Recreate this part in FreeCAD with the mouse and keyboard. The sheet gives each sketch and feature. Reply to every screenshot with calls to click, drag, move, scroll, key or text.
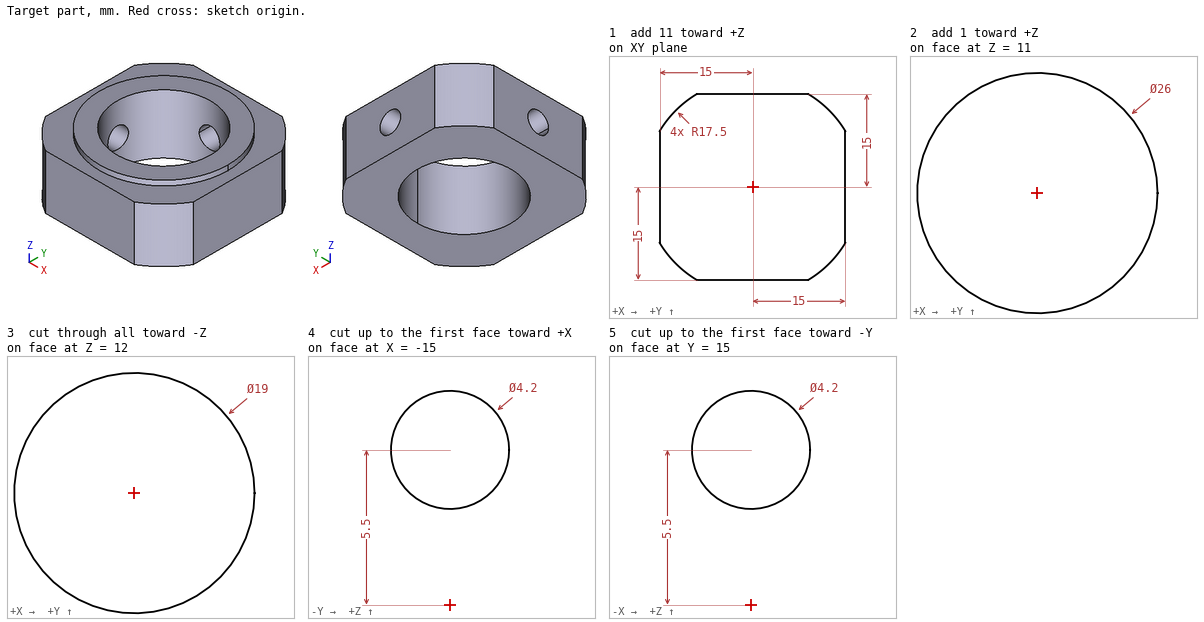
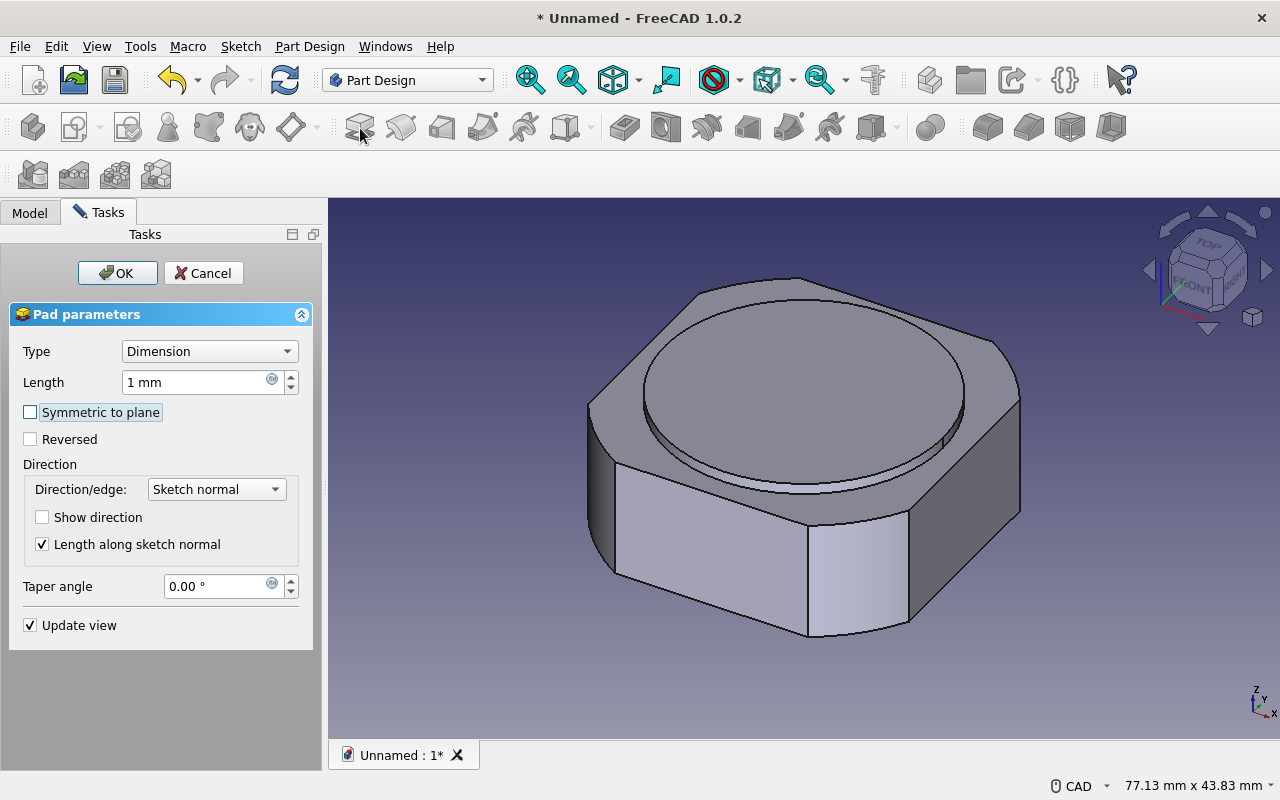
click(118, 273)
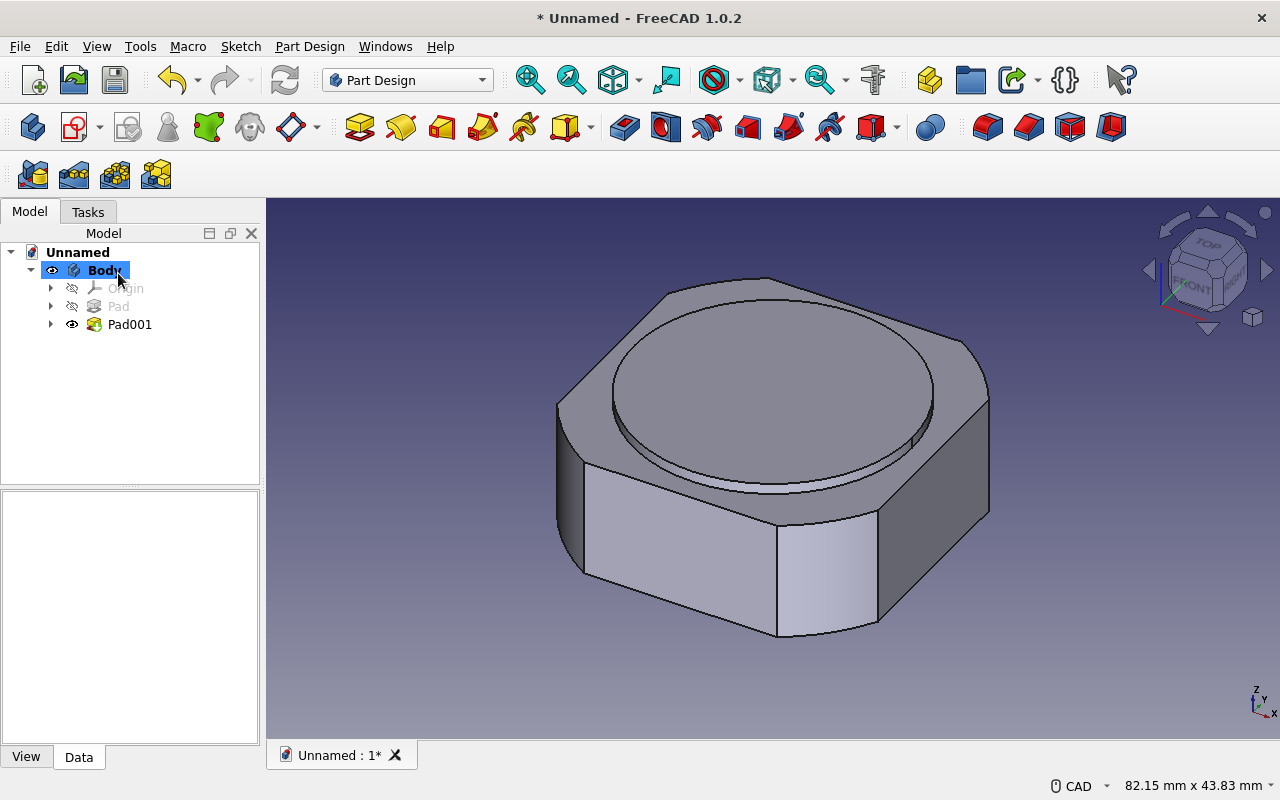
click(773, 391)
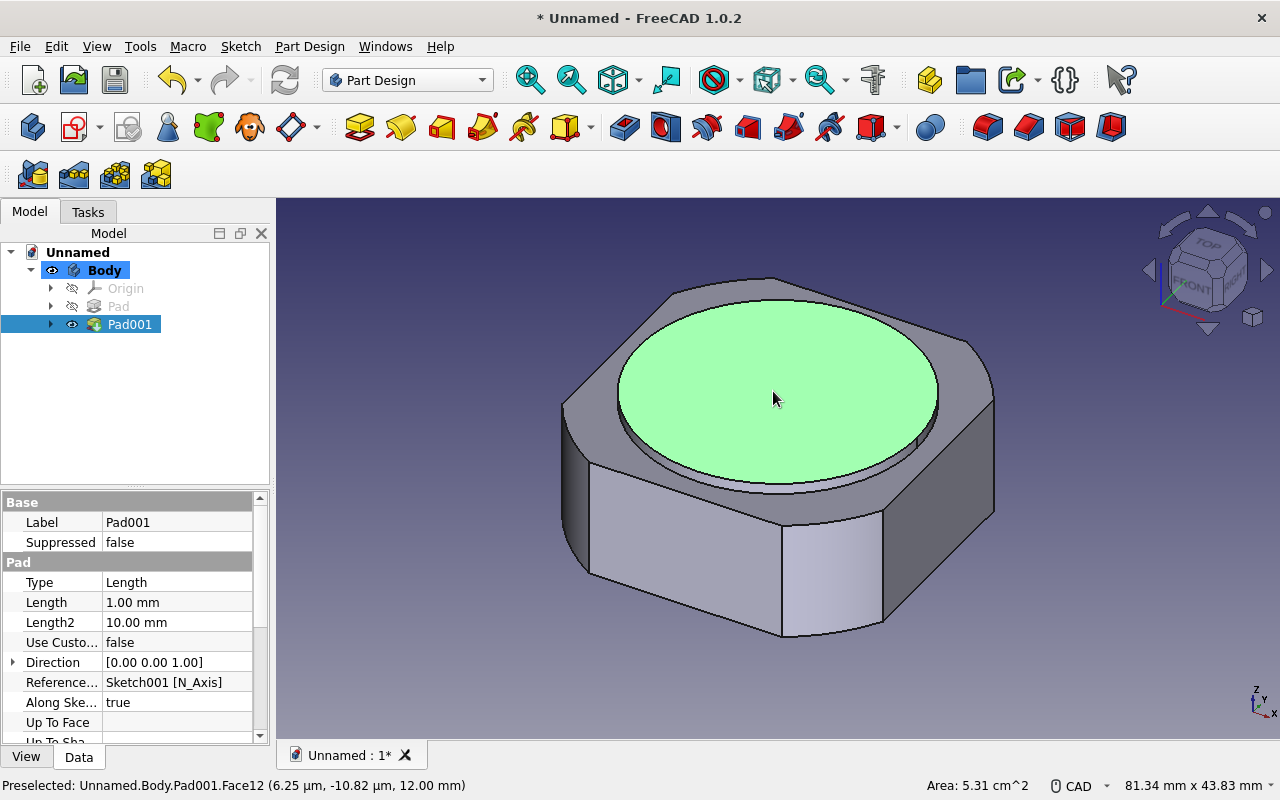
click(74, 128)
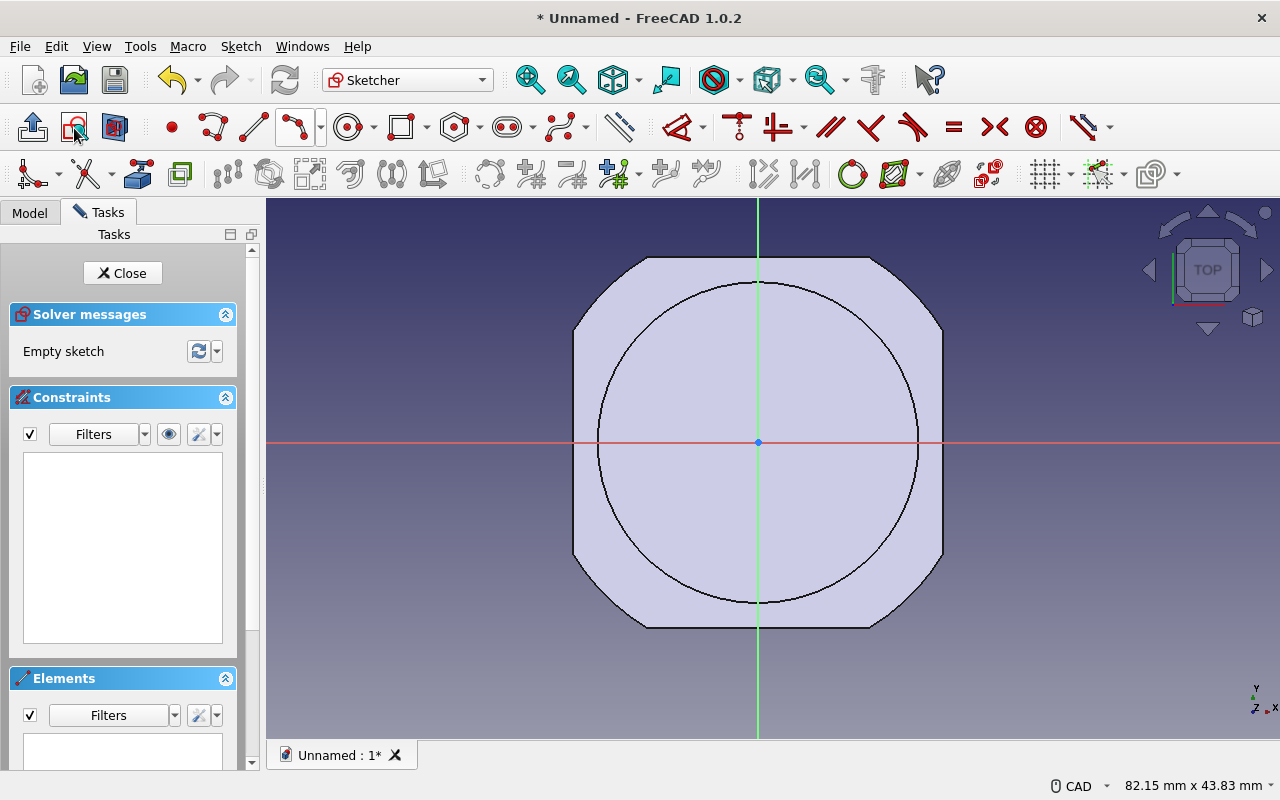
scroll(867, 390, up, 2)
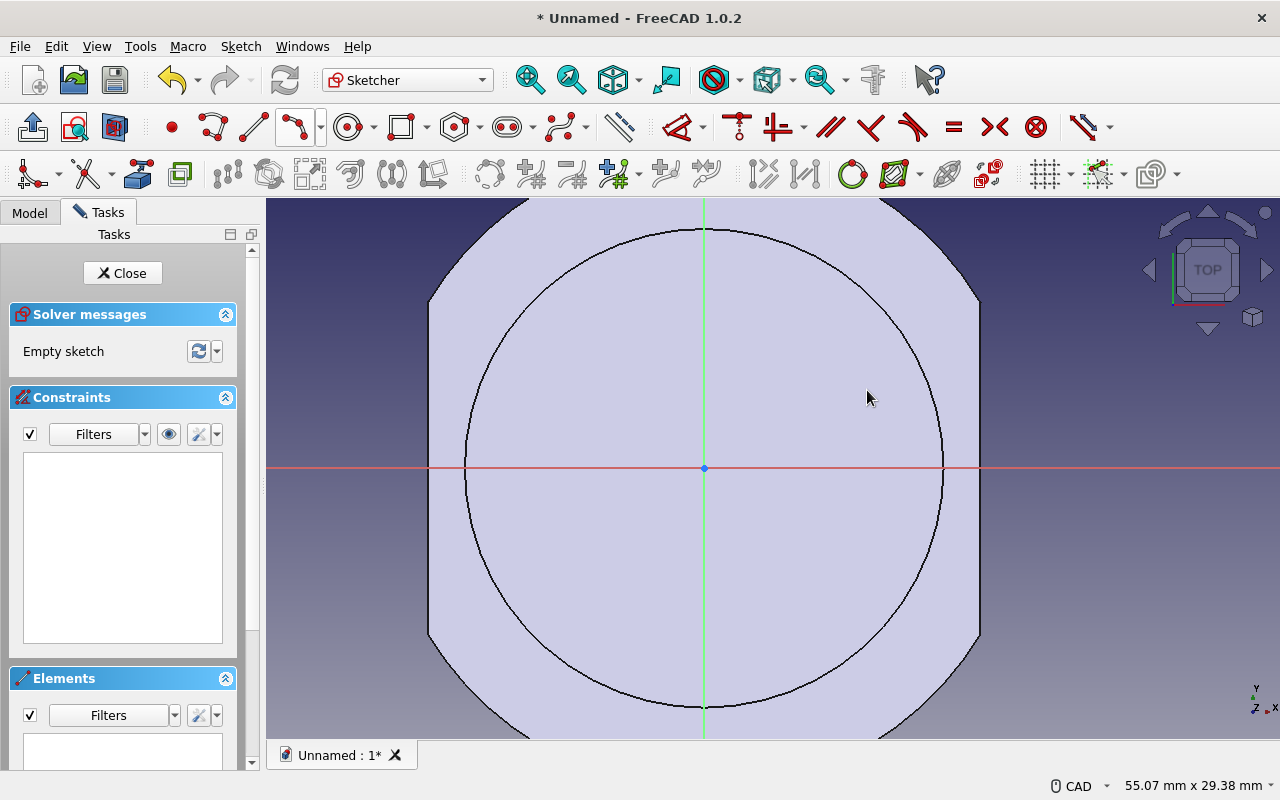
key(g)
key(c)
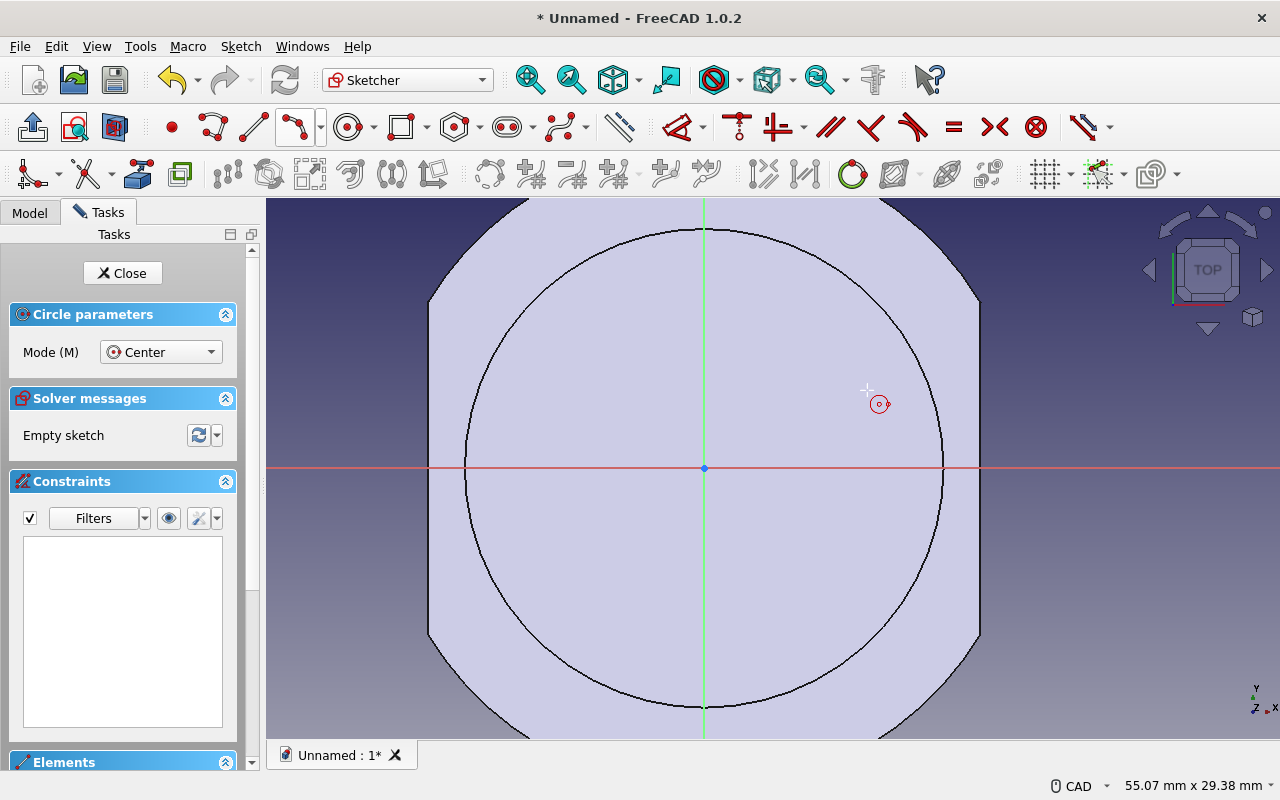
click(704, 468)
click(828, 345)
key(Escape)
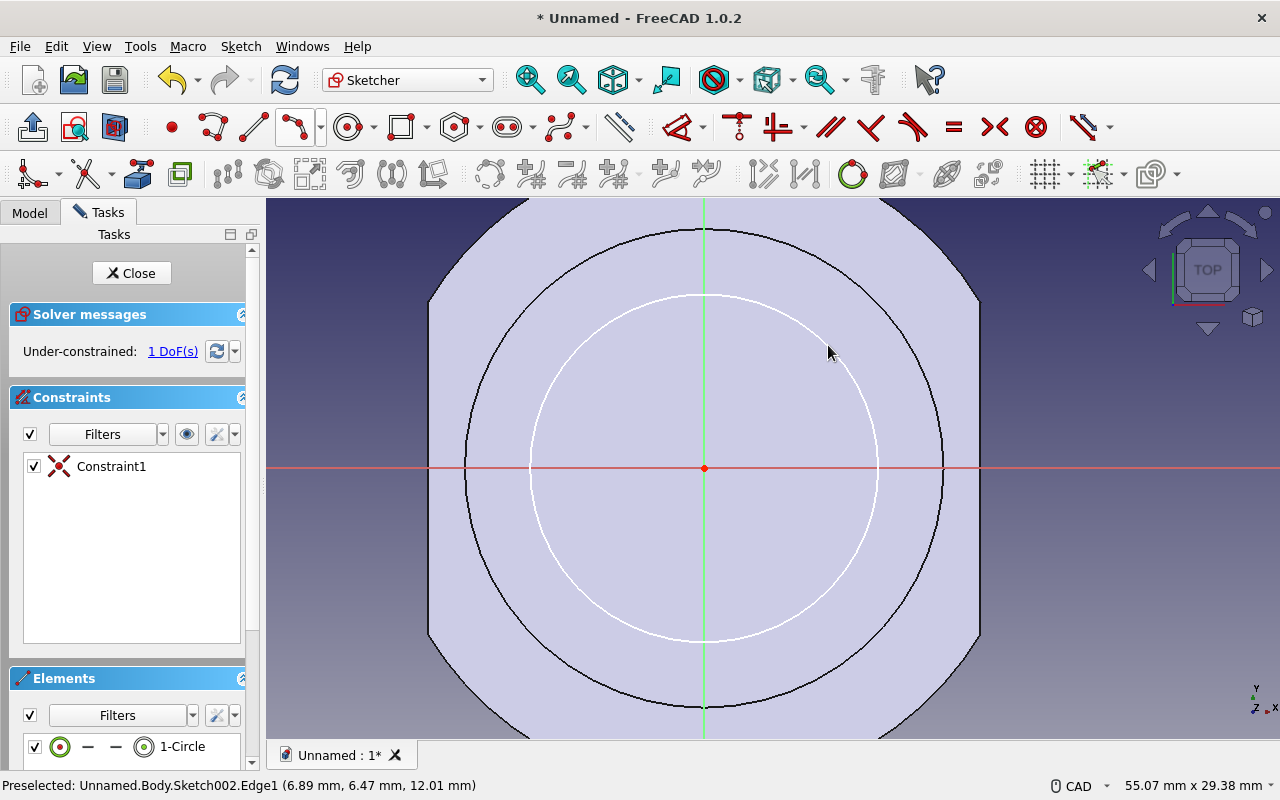
click(676, 128)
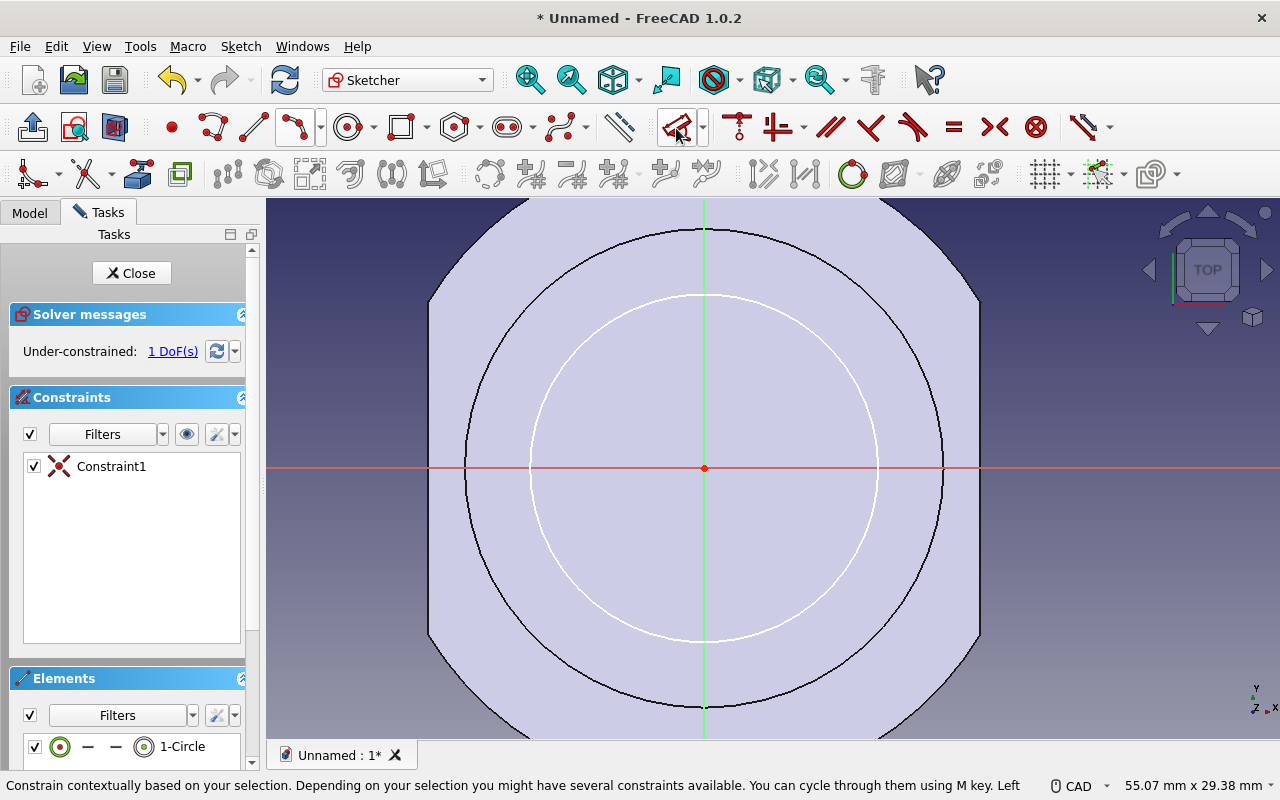
click(827, 345)
click(850, 322)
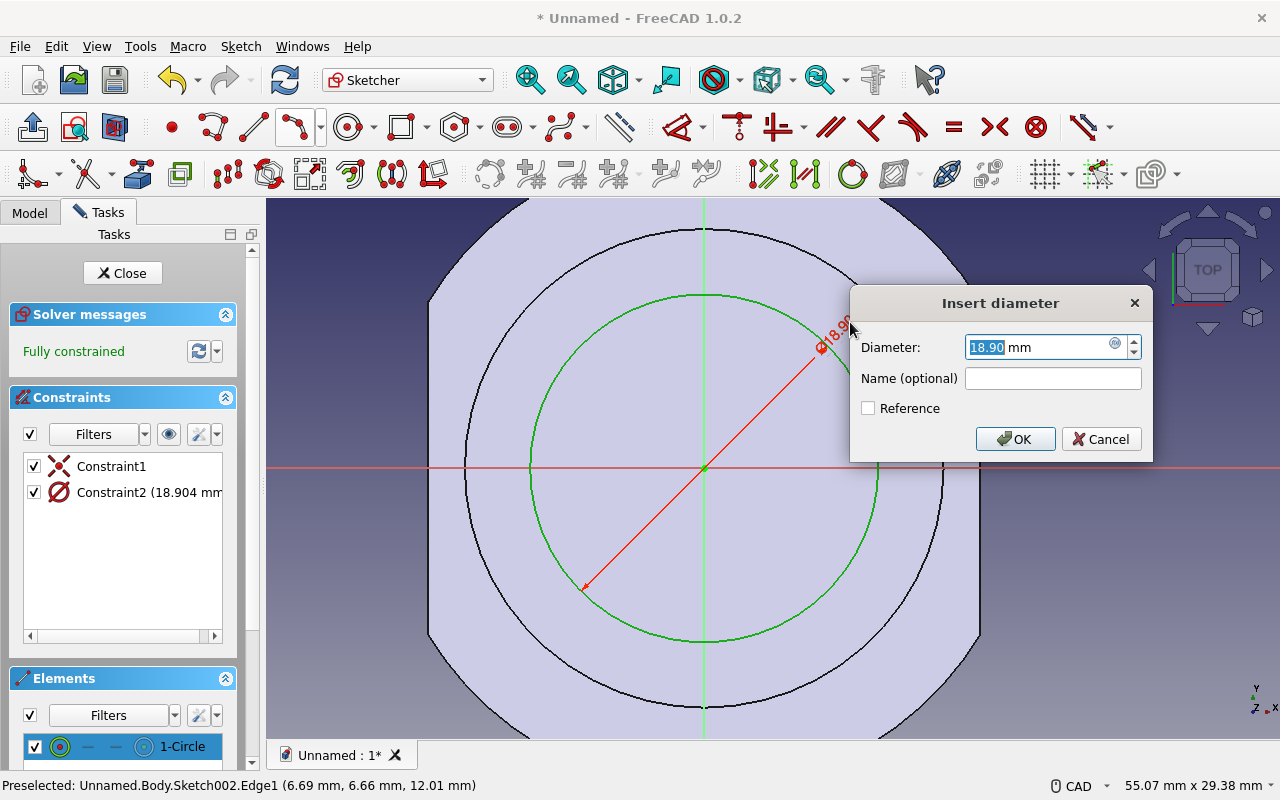
text(19)
key(Return)
key(Escape)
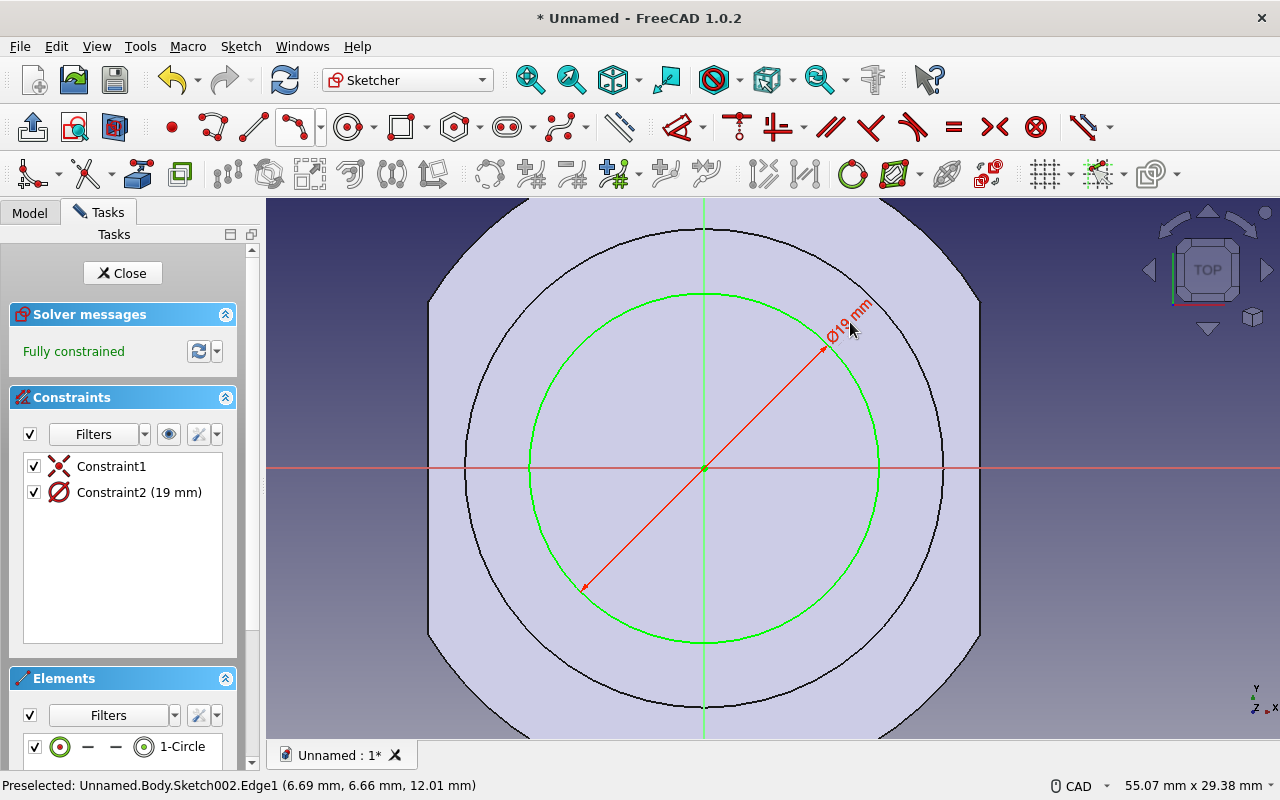
click(123, 273)